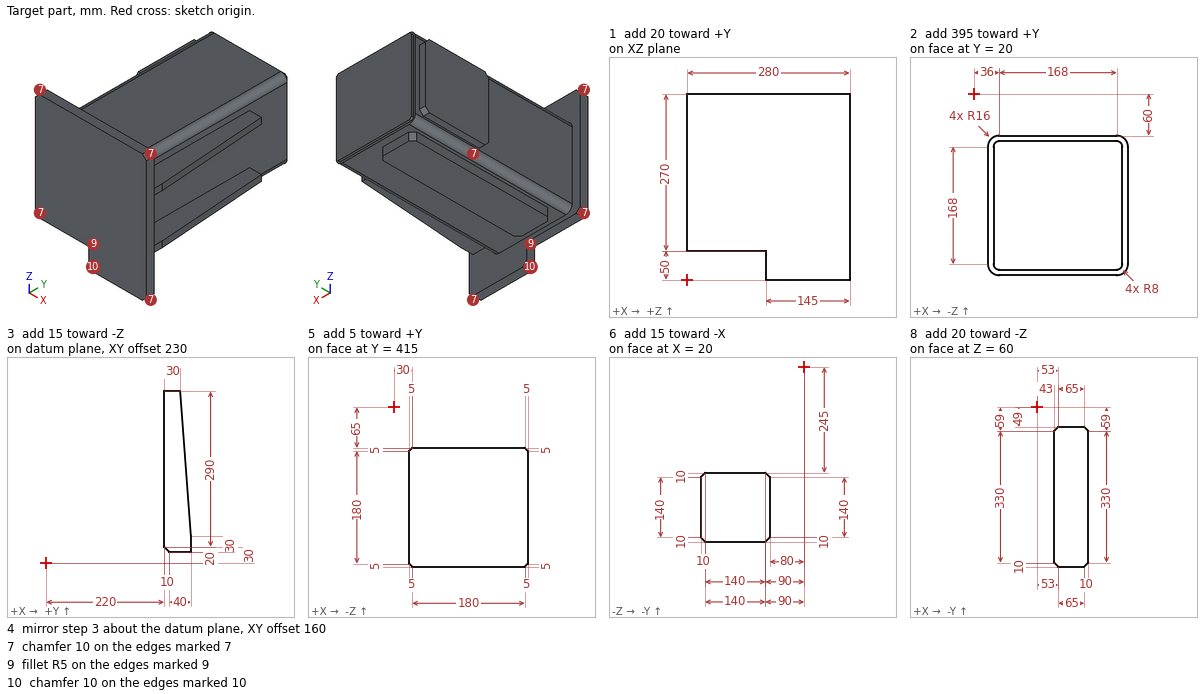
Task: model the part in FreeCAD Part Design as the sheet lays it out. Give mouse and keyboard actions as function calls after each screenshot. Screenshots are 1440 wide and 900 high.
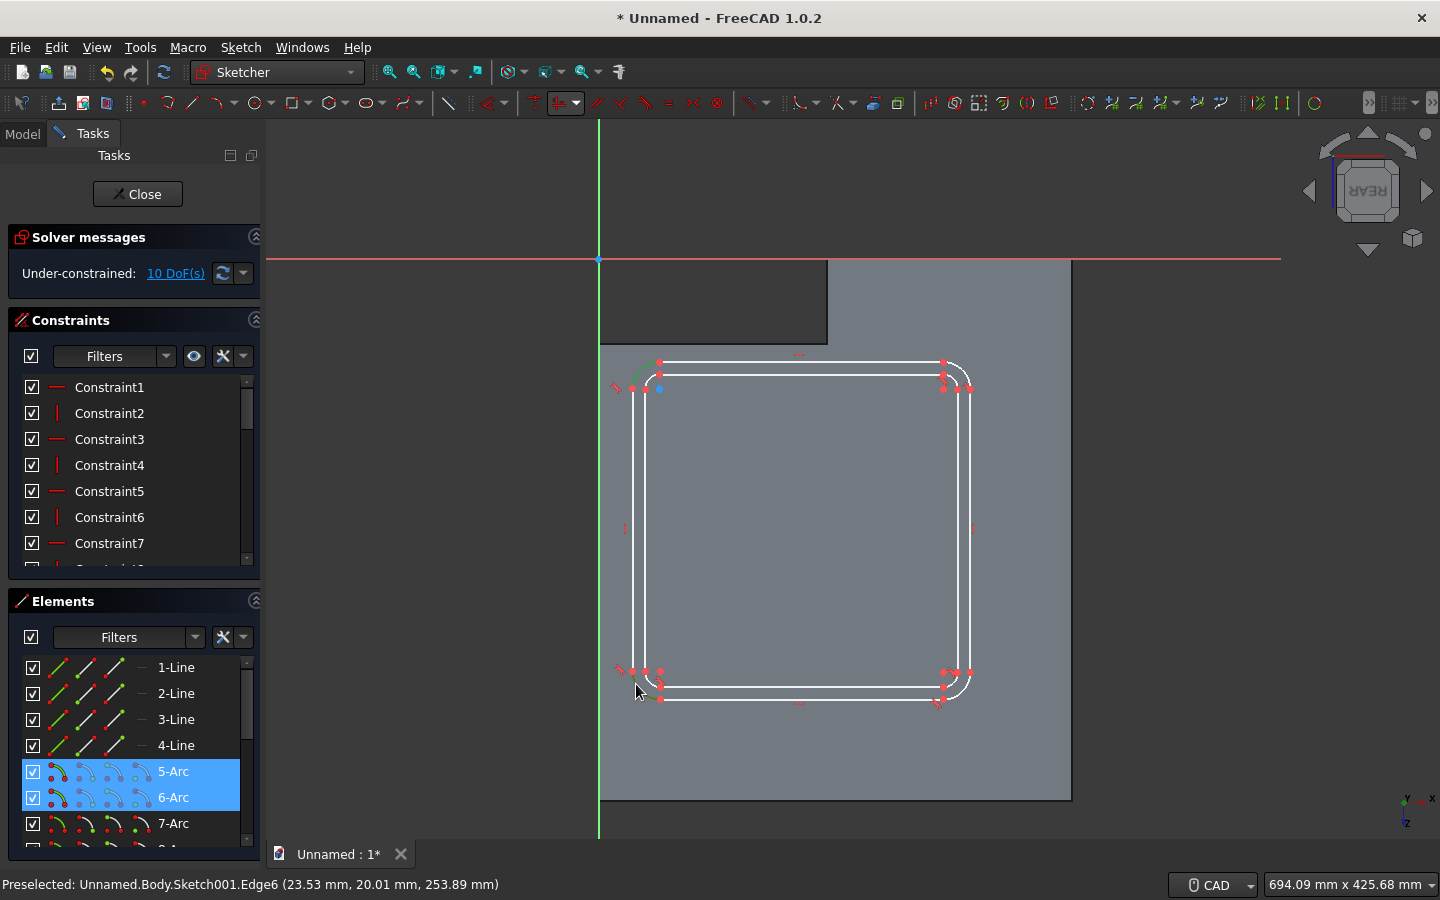
click(967, 685)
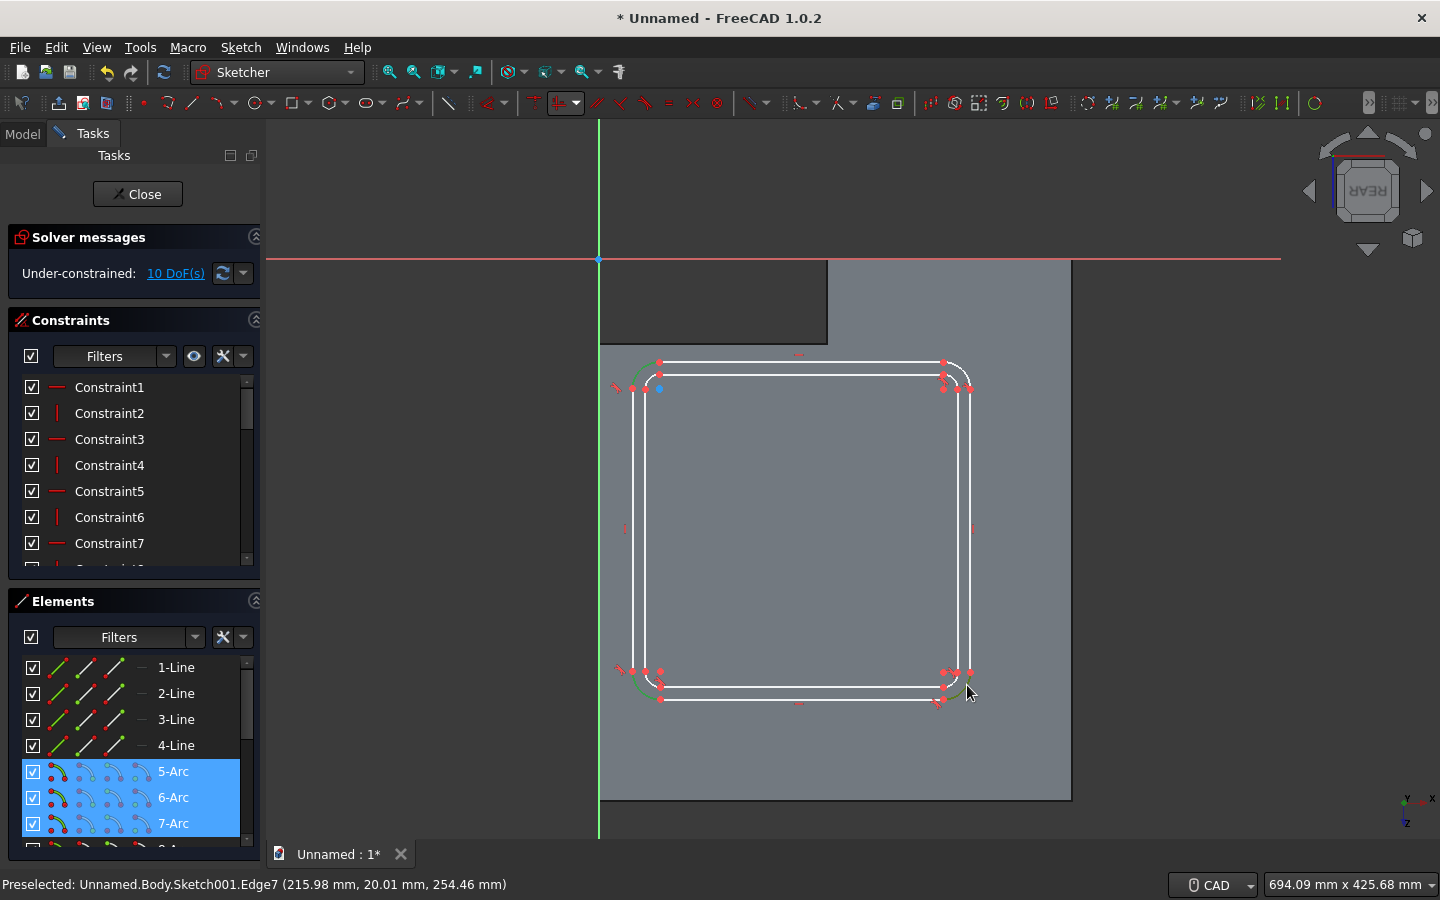
click(967, 377)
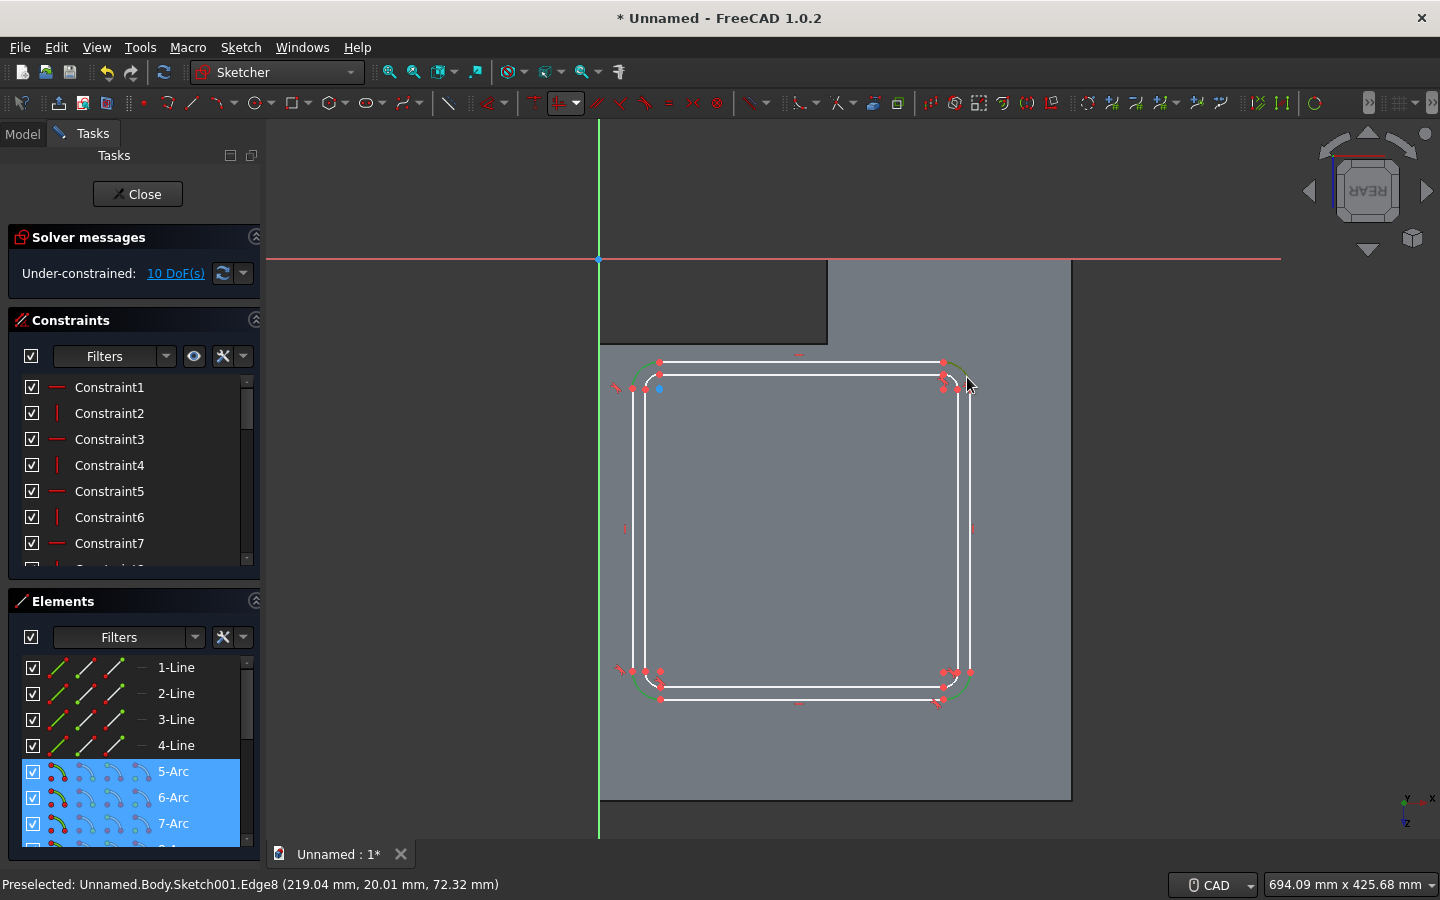
click(670, 104)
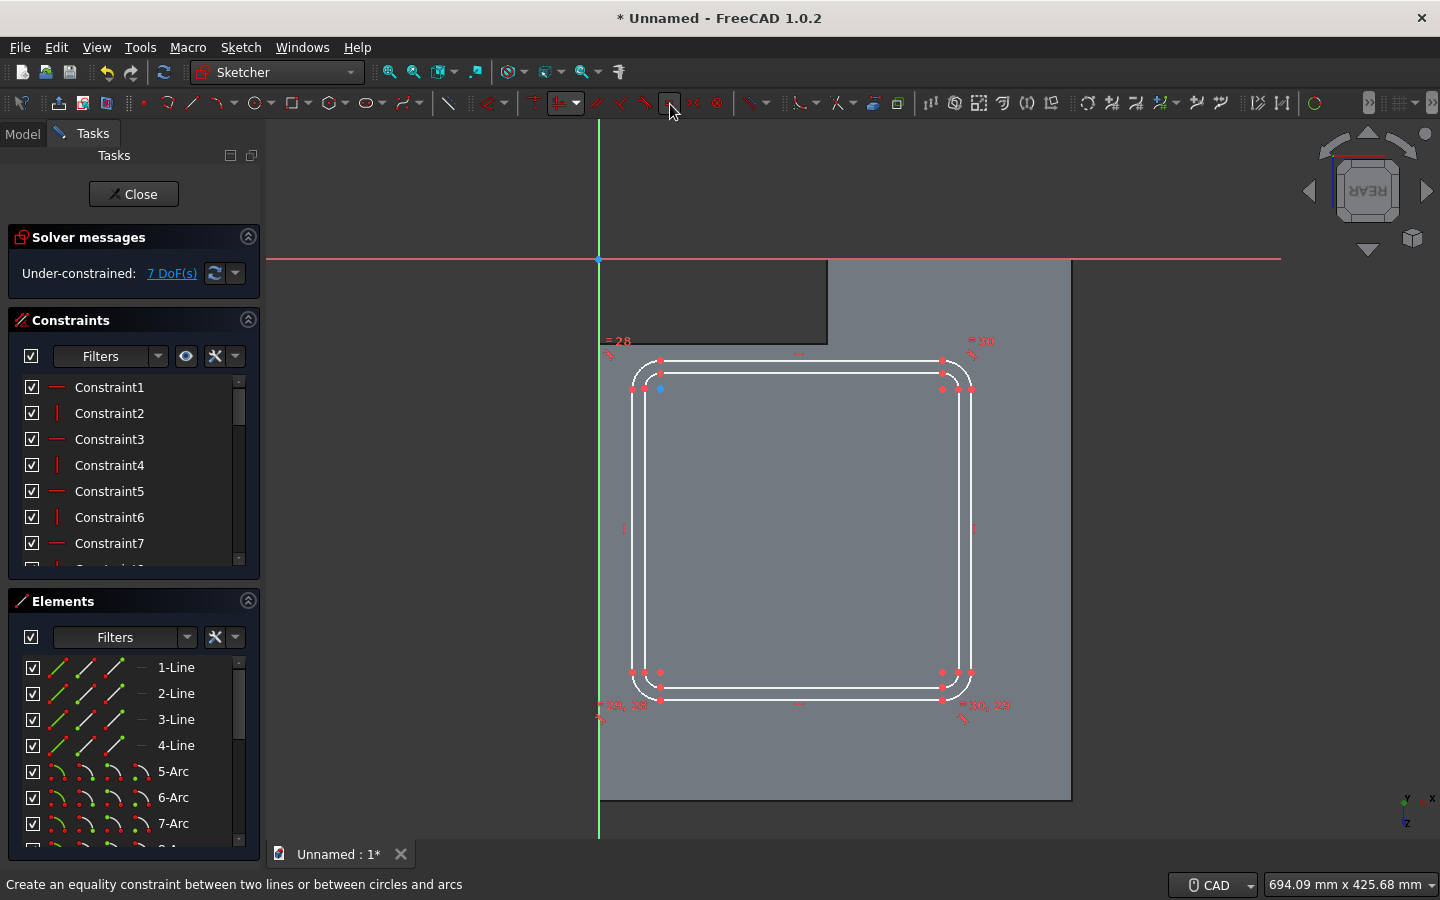
click(954, 378)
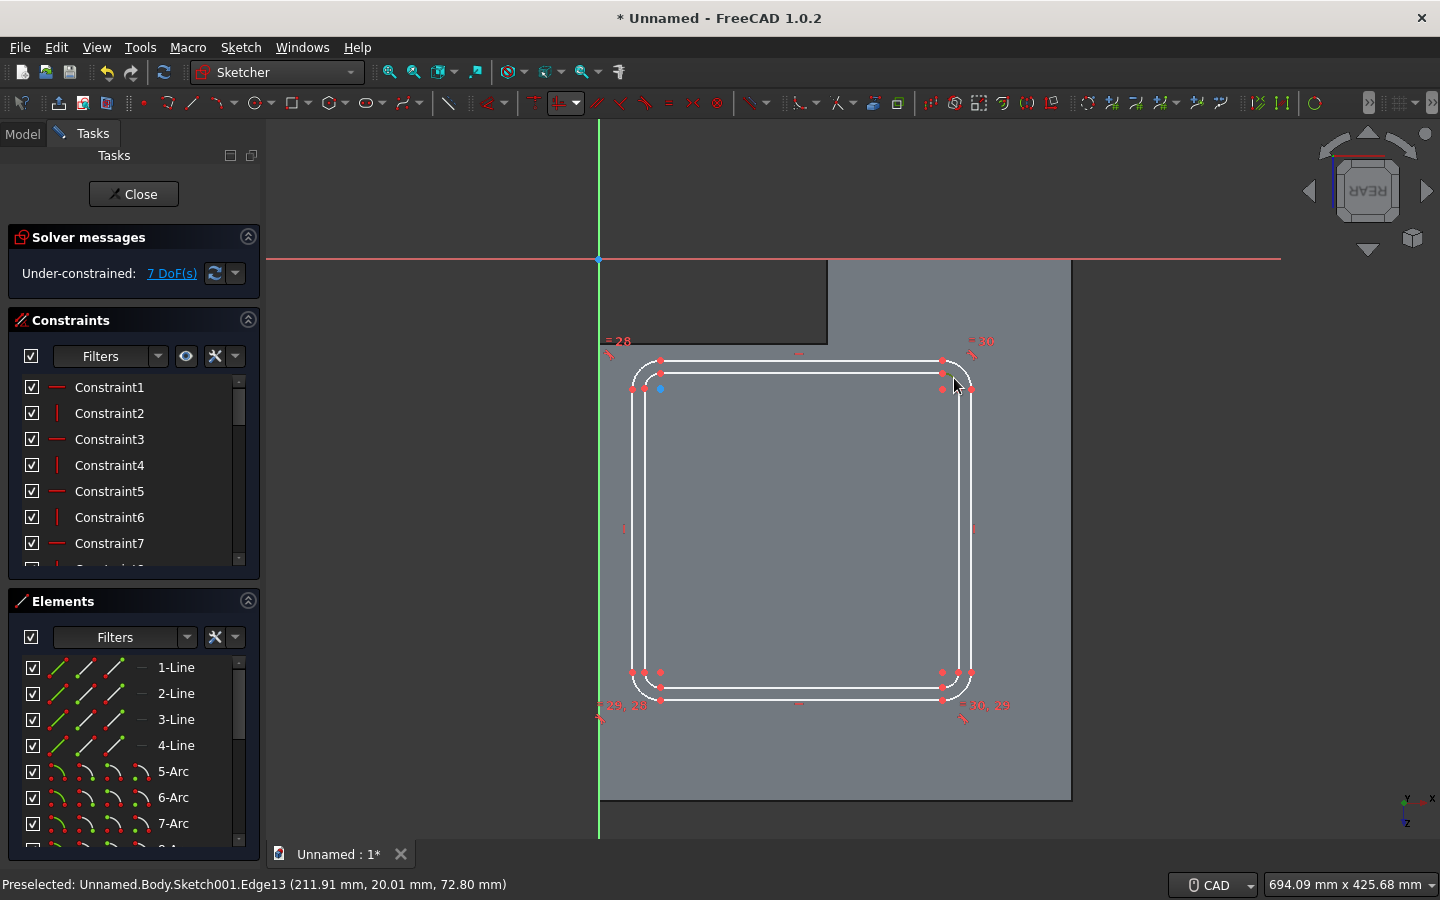
click(649, 378)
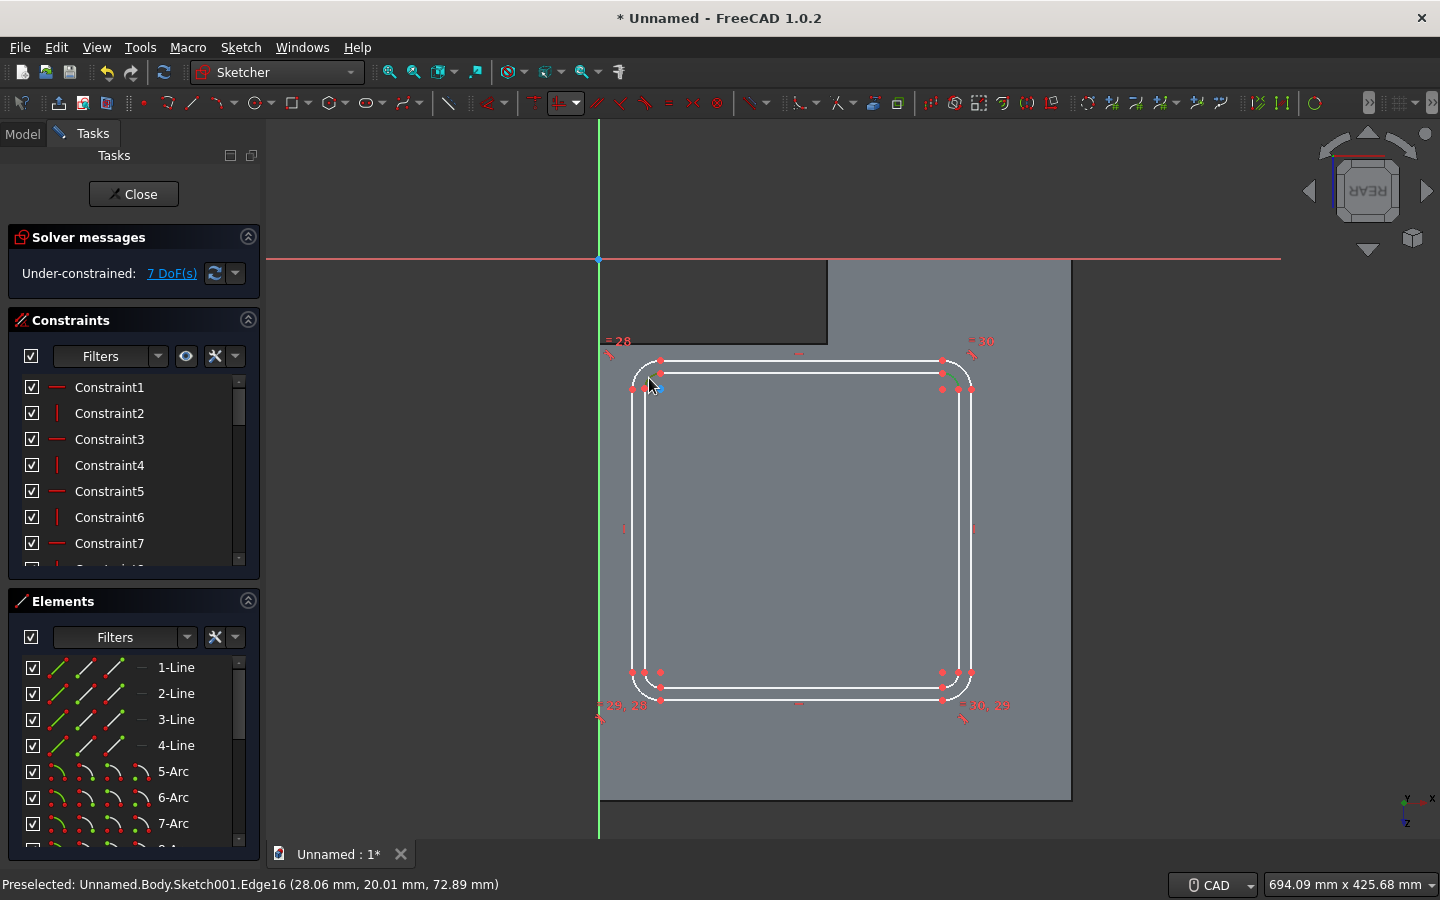
click(670, 104)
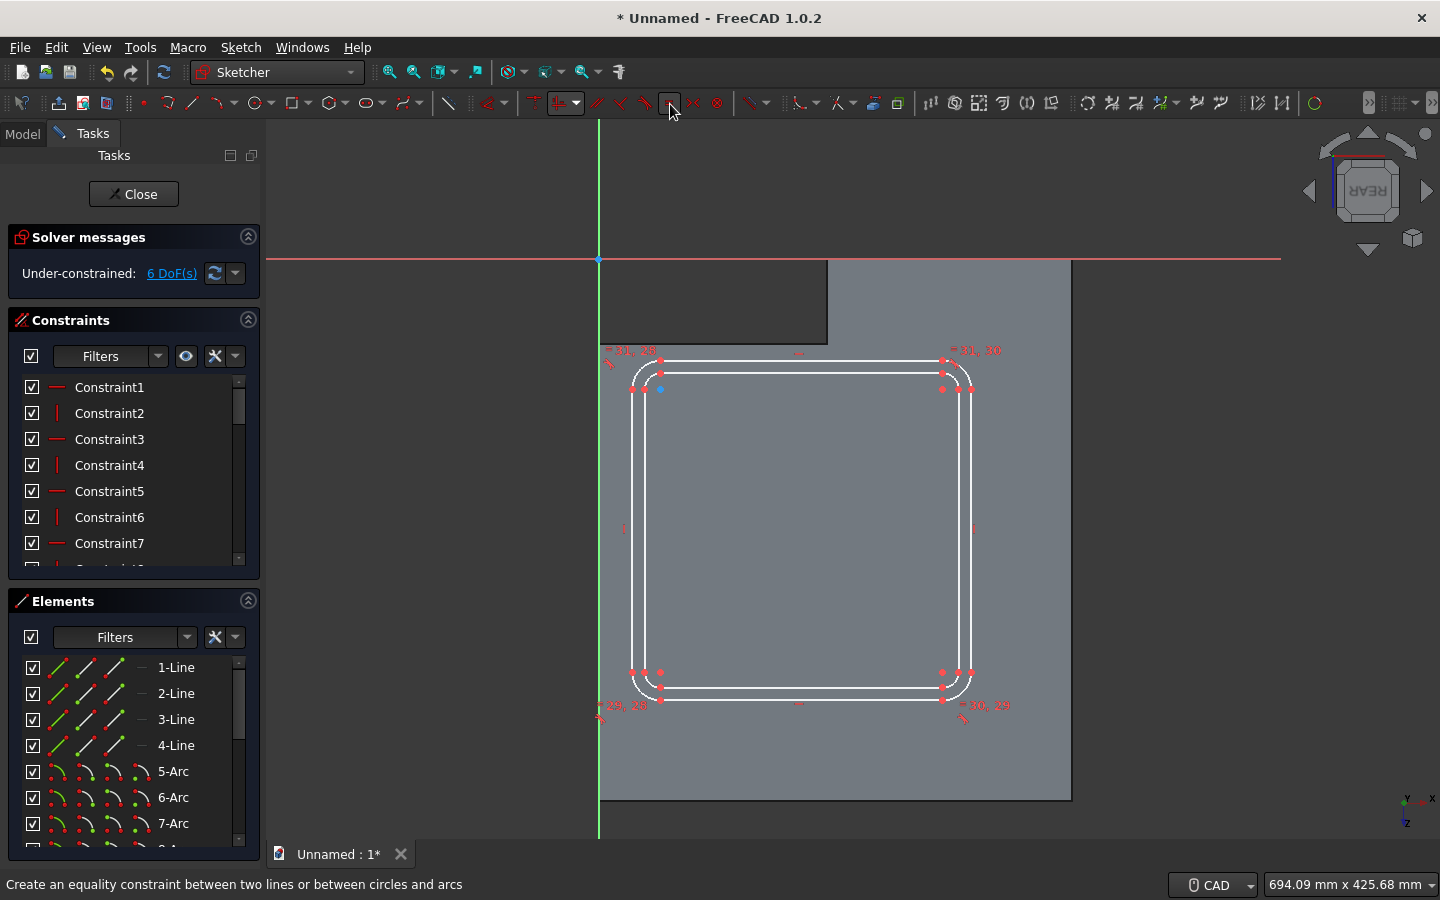
click(488, 104)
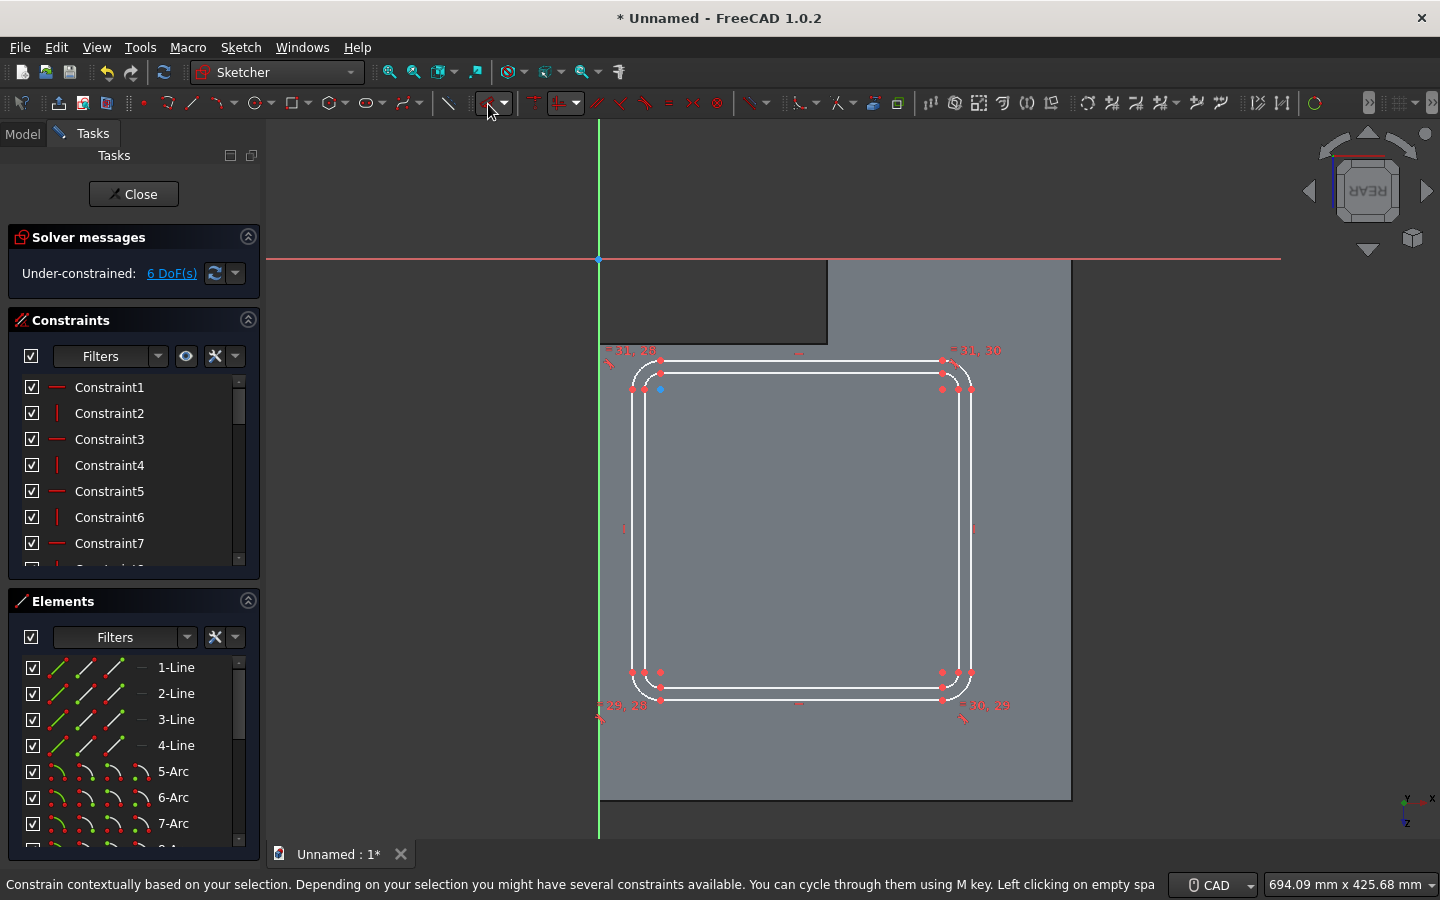
scroll(648, 364, up, 2)